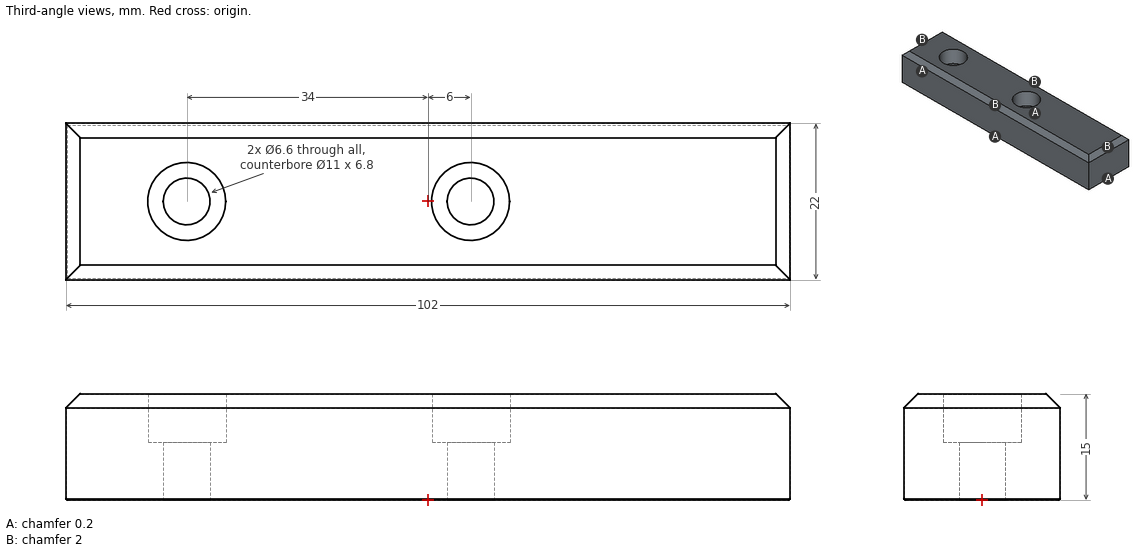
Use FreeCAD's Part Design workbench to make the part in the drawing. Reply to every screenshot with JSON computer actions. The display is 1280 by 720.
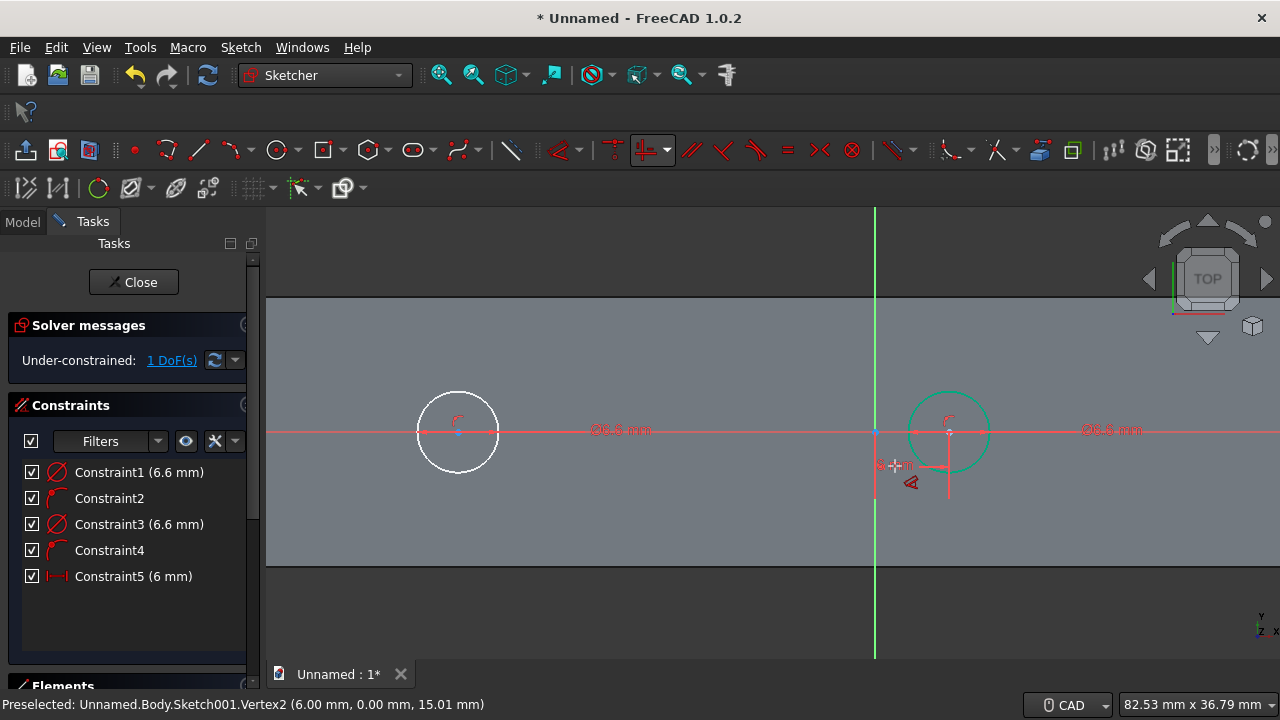
{"action": "left_click", "coordinate": [458, 432]}
{"action": "left_click", "coordinate": [667, 466]}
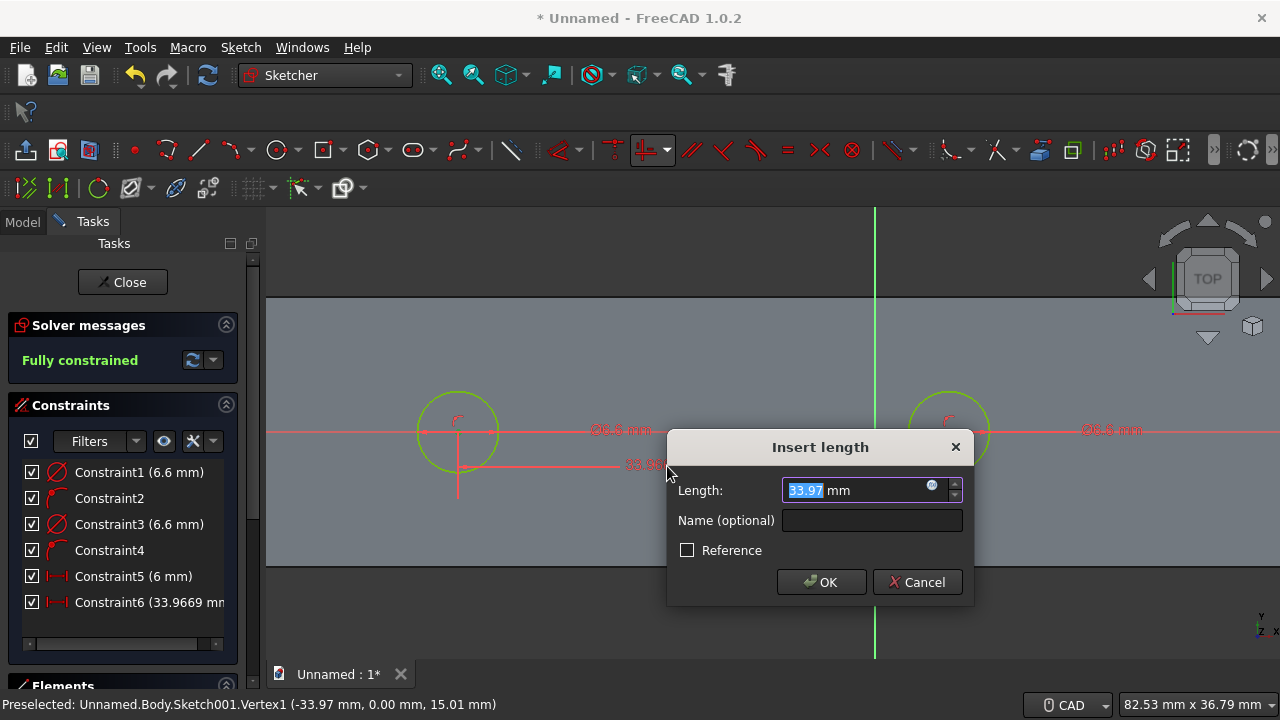
{"action": "type", "text": "34"}
{"action": "key", "text": "Return"}
{"action": "key", "text": "Escape"}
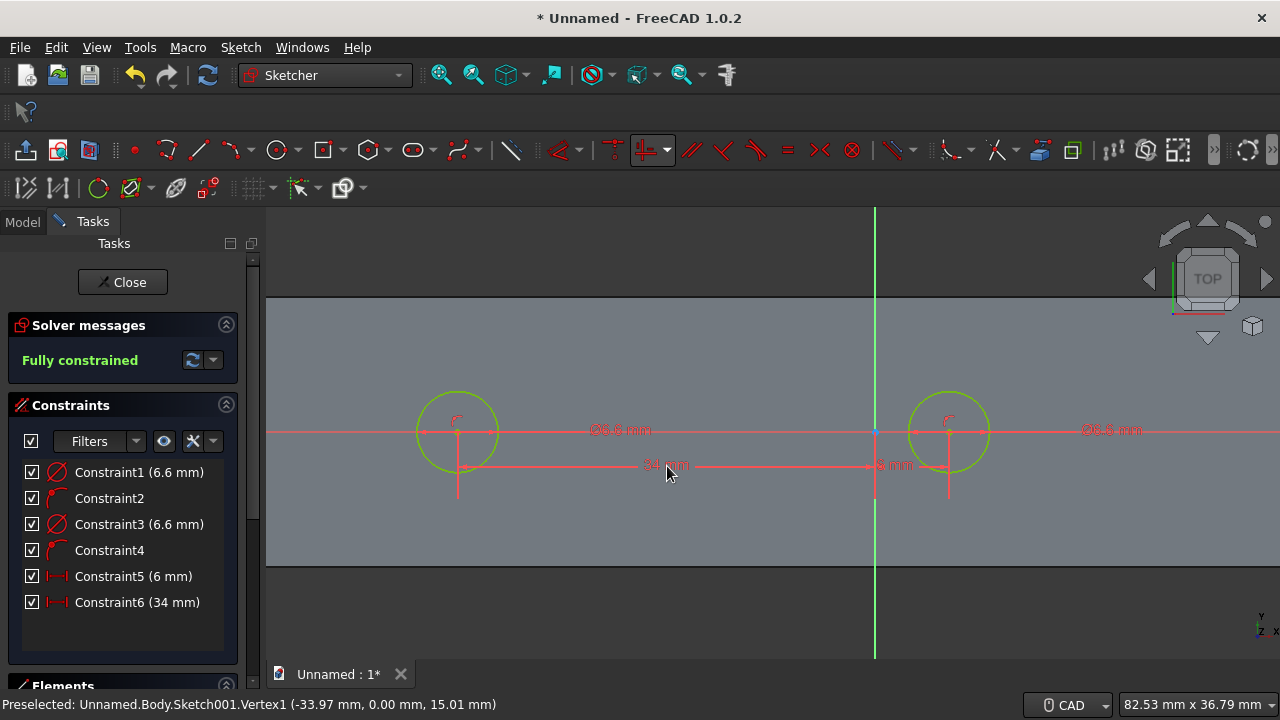
{"action": "left_click", "coordinate": [123, 282]}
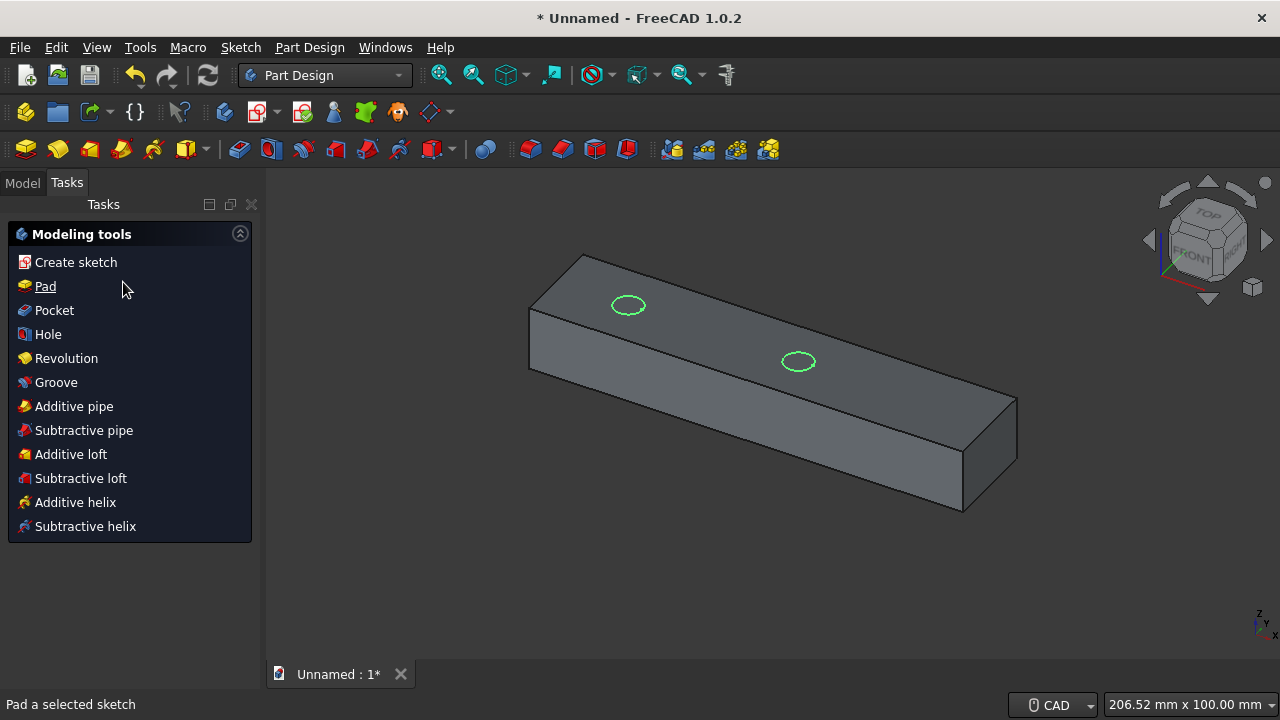
{"action": "left_click", "coordinate": [272, 150]}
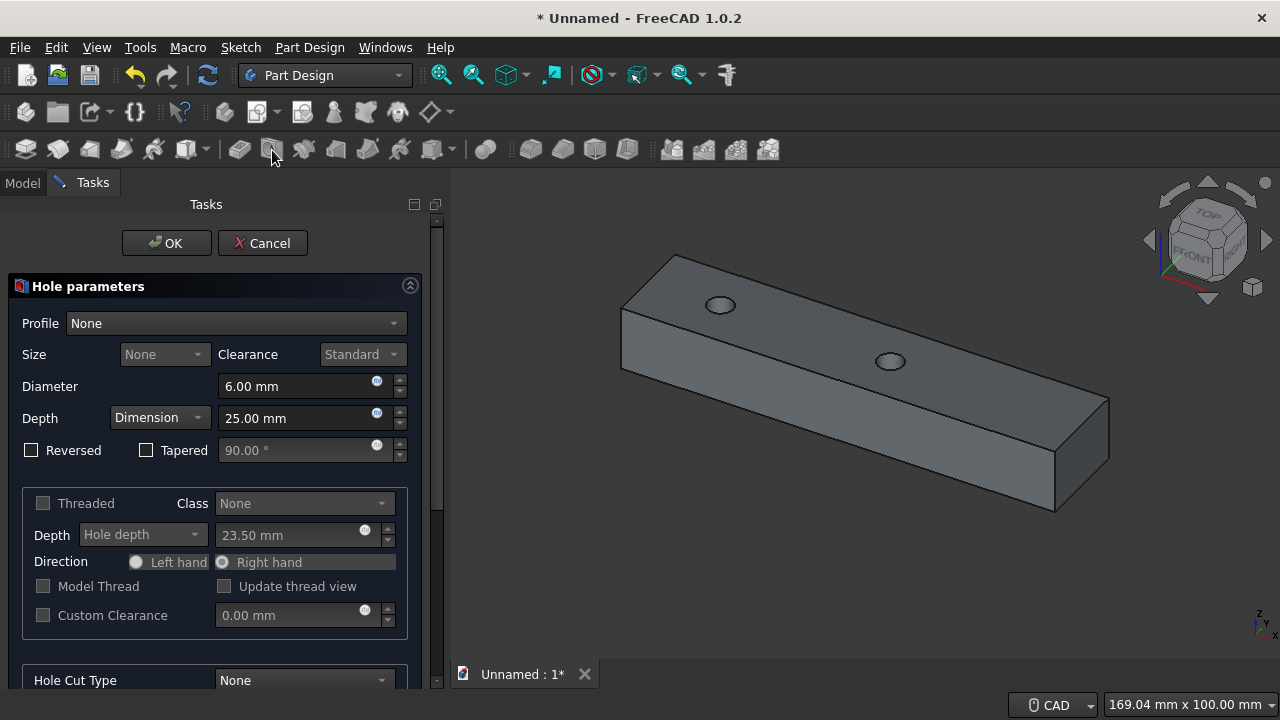
{"action": "triple_click", "coordinate": [305, 386]}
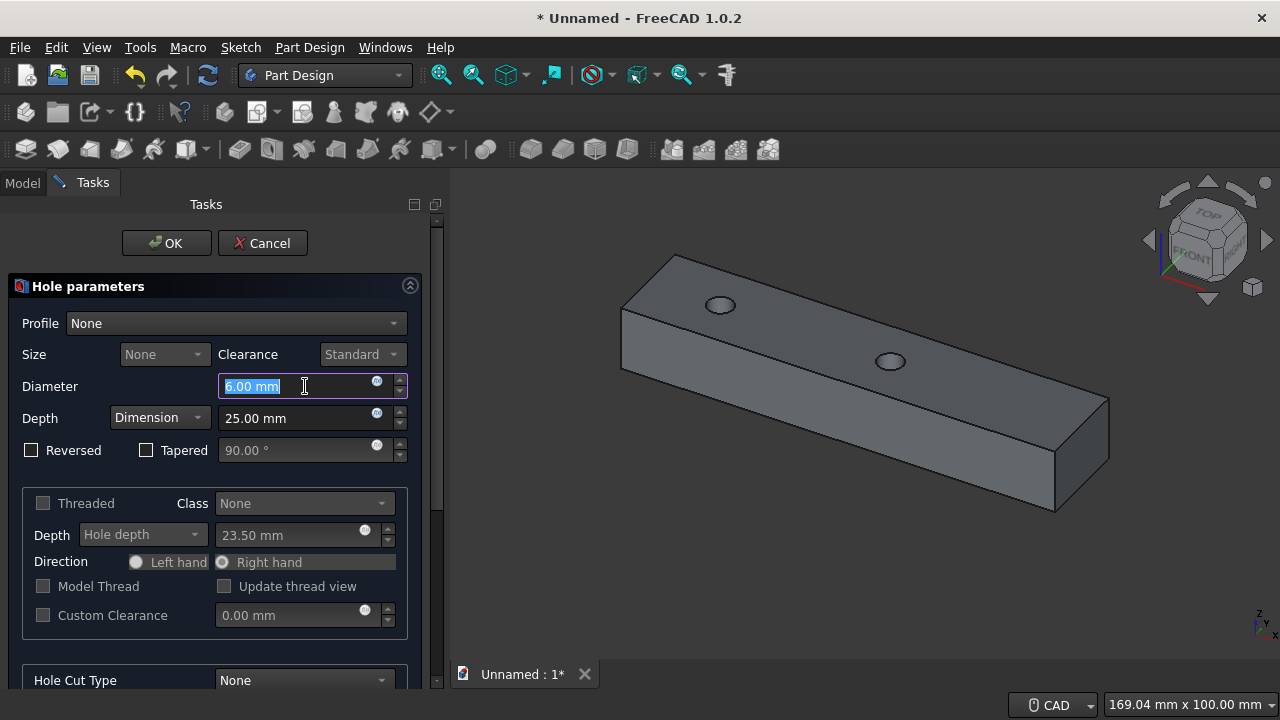
{"action": "type", "text": "6.6"}
{"action": "key", "text": "Tab"}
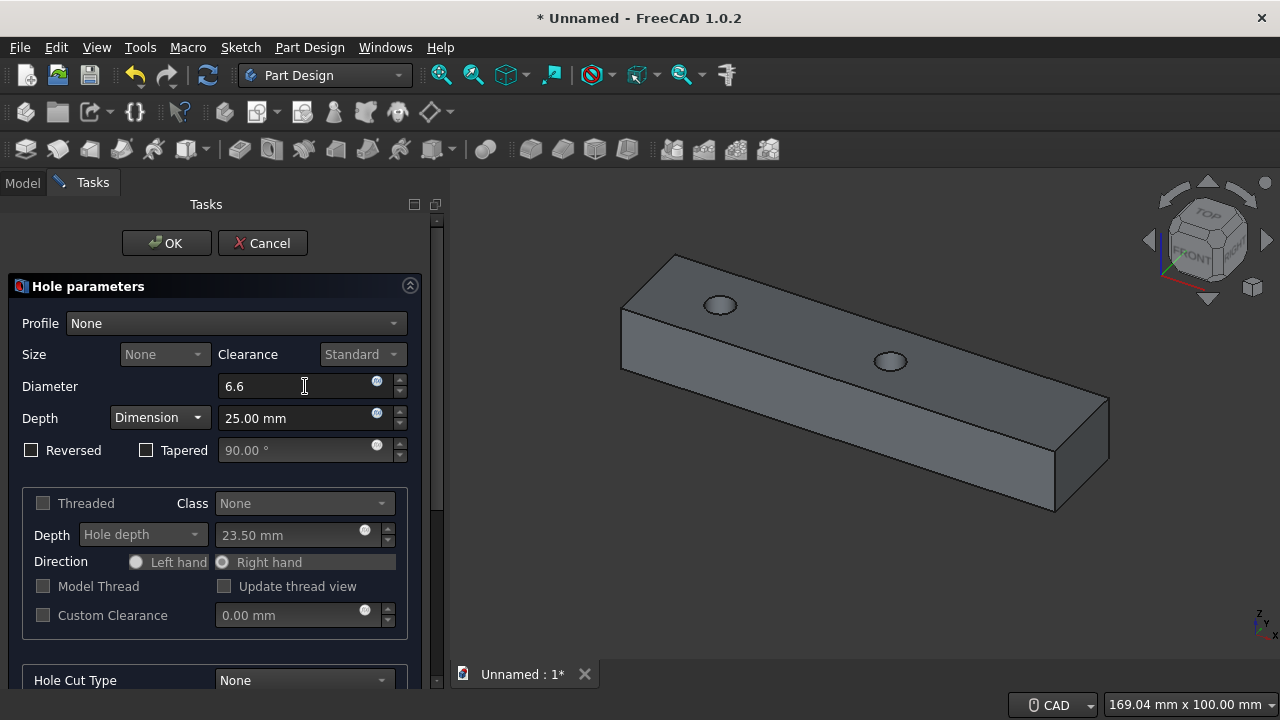
{"action": "left_click", "coordinate": [161, 418]}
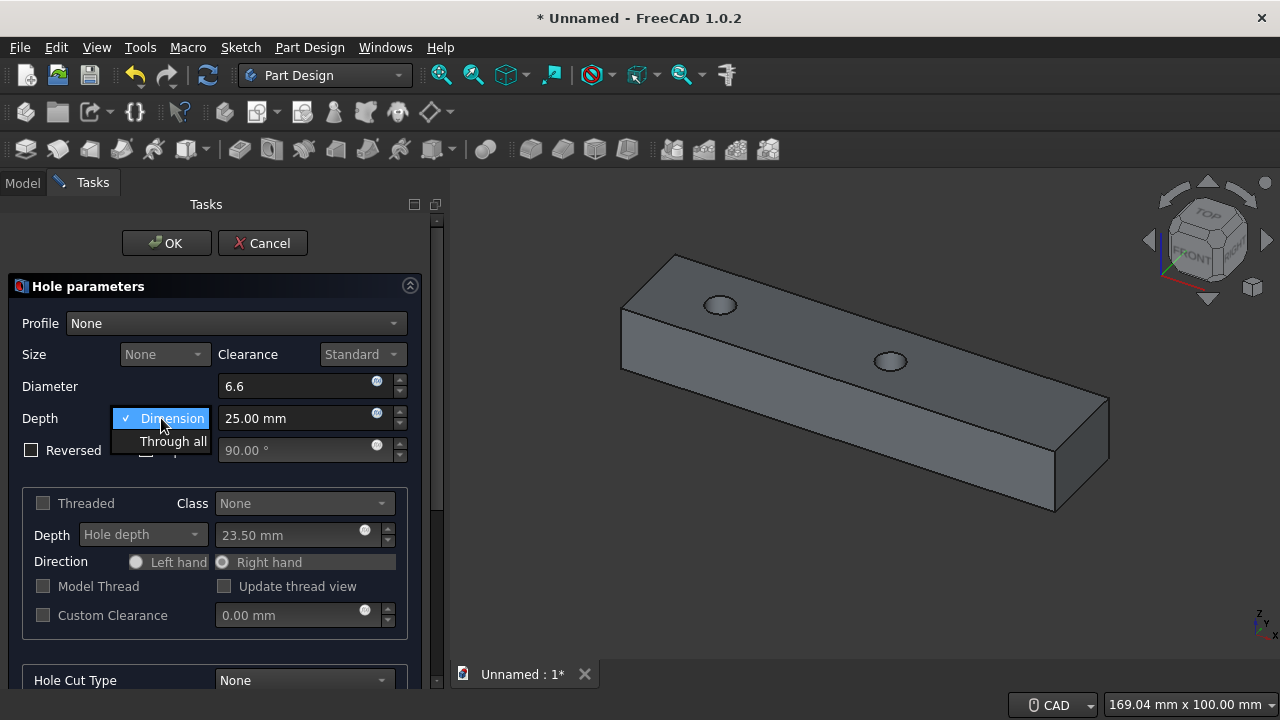
{"action": "left_click", "coordinate": [160, 442]}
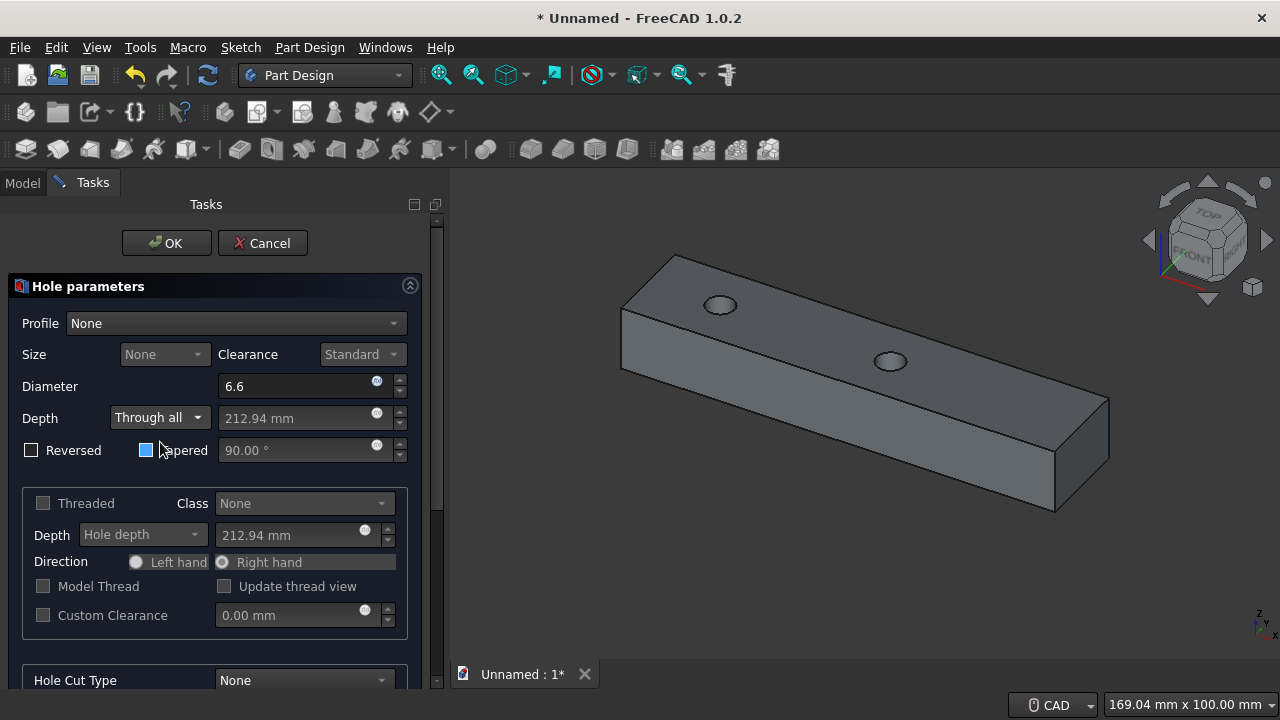
{"action": "scroll", "coordinate": [437, 451], "scroll_direction": "down", "scroll_amount": 2}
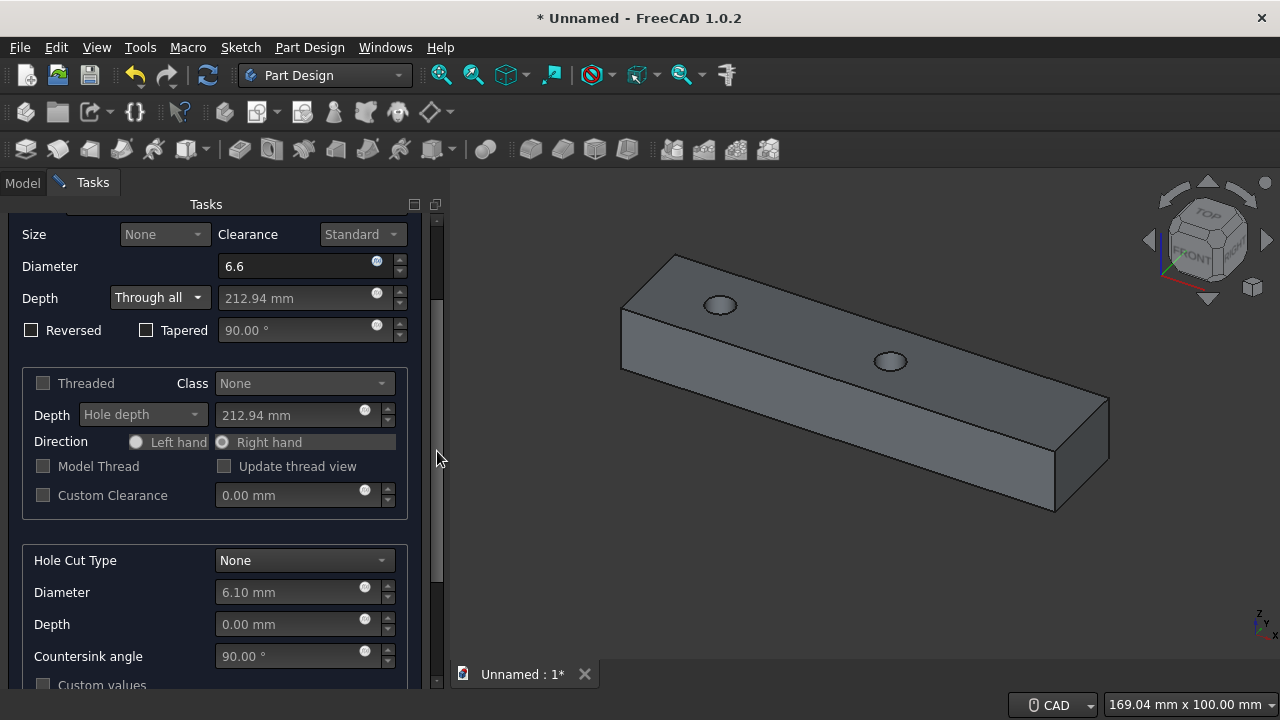
{"action": "left_click", "coordinate": [306, 560]}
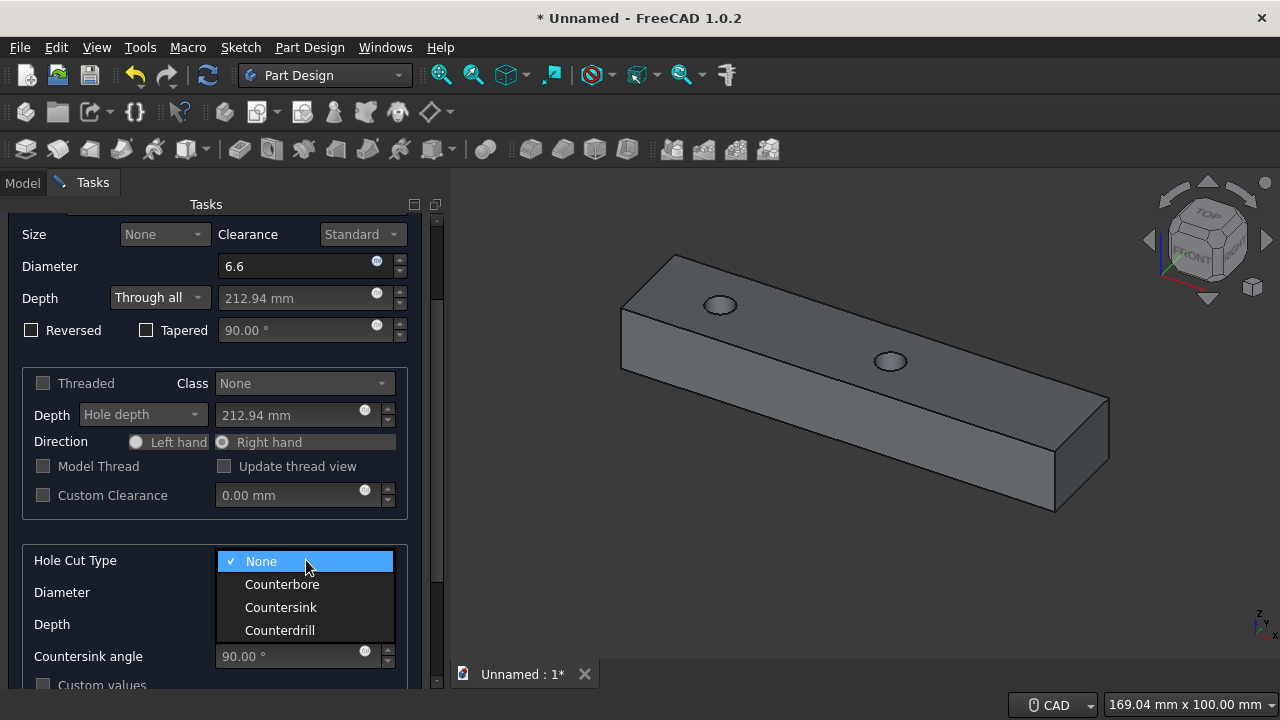
{"action": "left_click", "coordinate": [304, 584]}